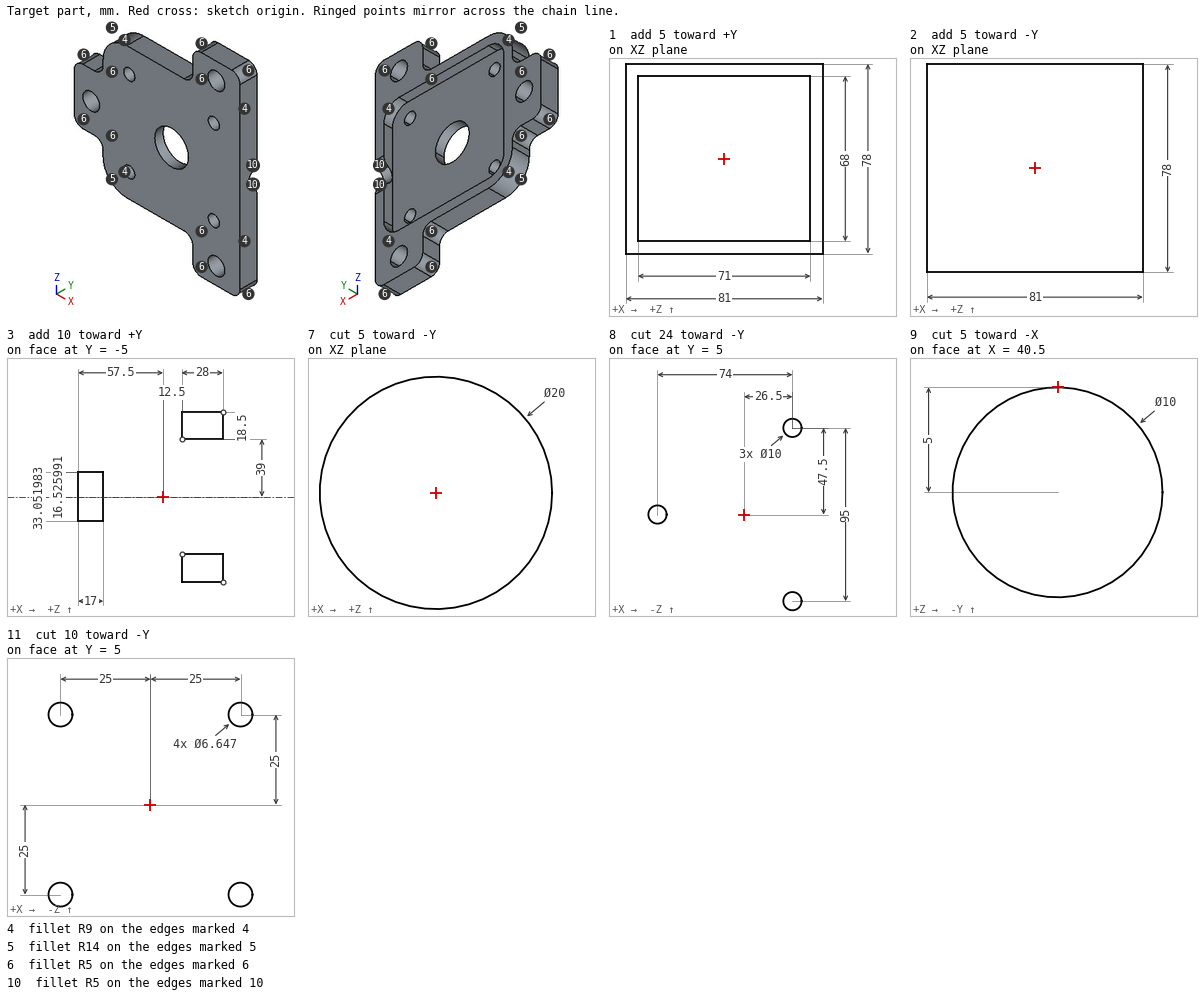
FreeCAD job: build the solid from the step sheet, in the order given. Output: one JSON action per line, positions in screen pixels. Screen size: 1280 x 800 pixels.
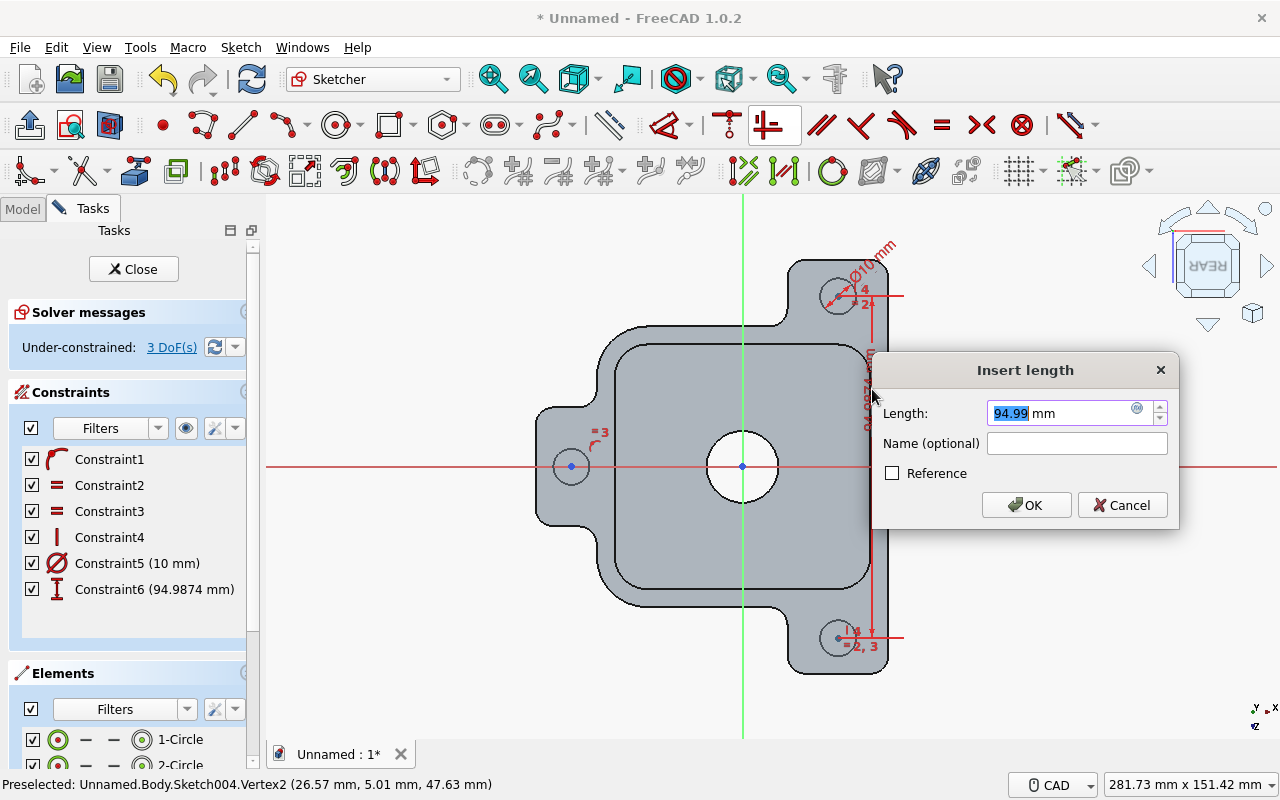
{"action": "type", "text": "95"}
{"action": "key", "text": "Return"}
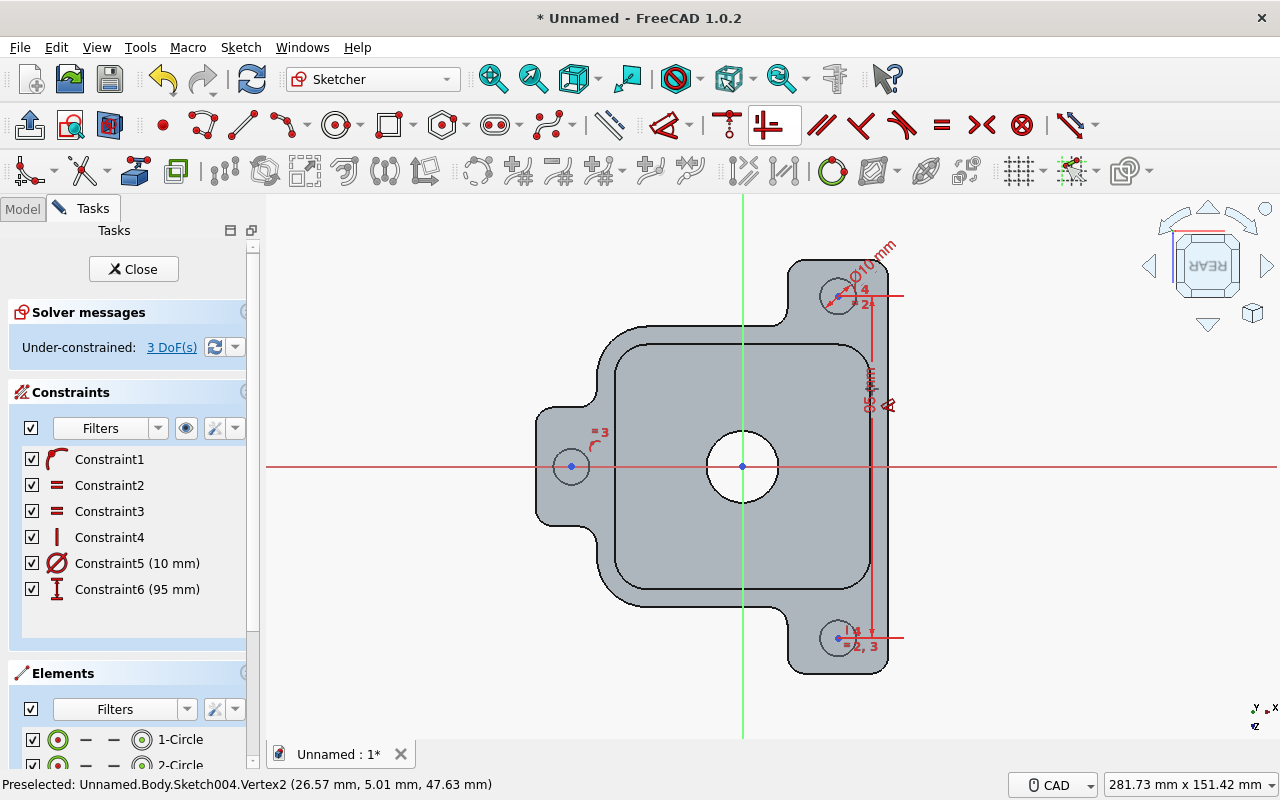
{"action": "left_click", "coordinate": [838, 296]}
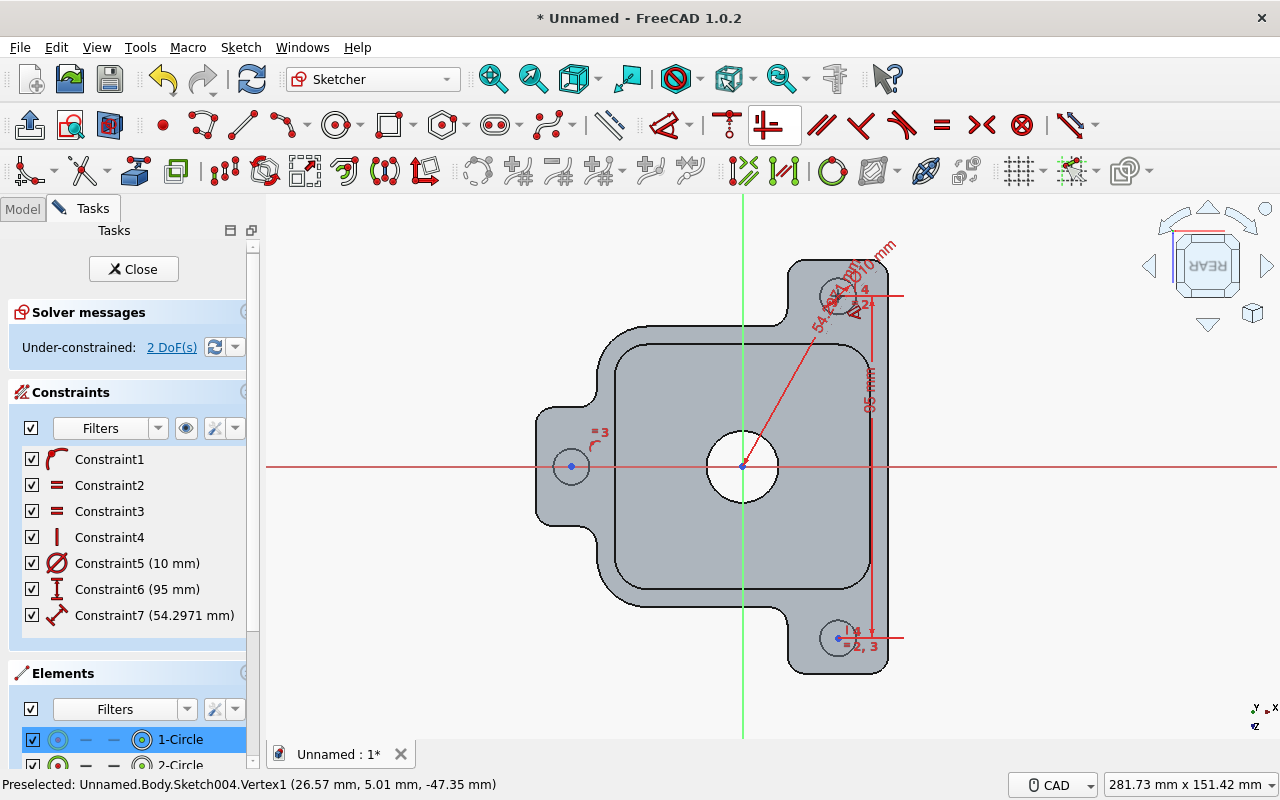
{"action": "left_click", "coordinate": [571, 467]}
{"action": "left_click", "coordinate": [705, 262]}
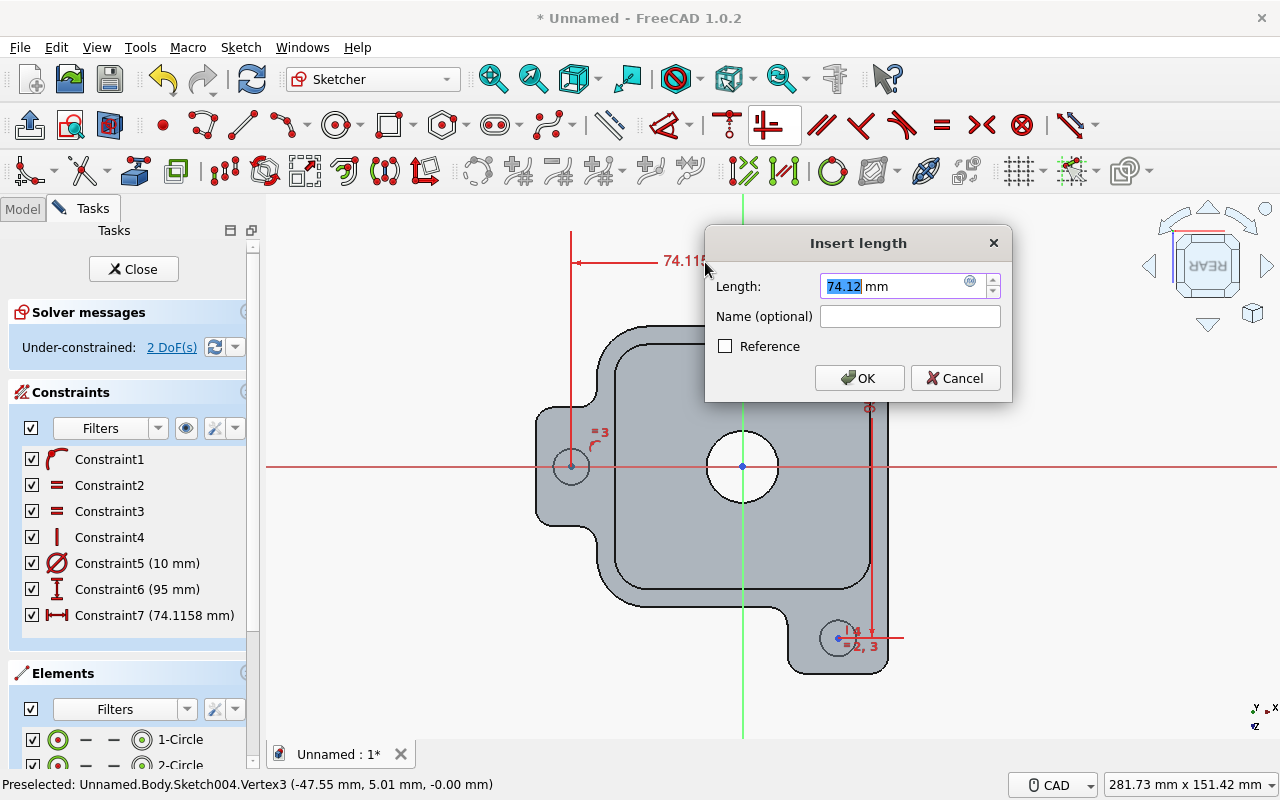
{"action": "type", "text": "74"}
{"action": "key", "text": "Return"}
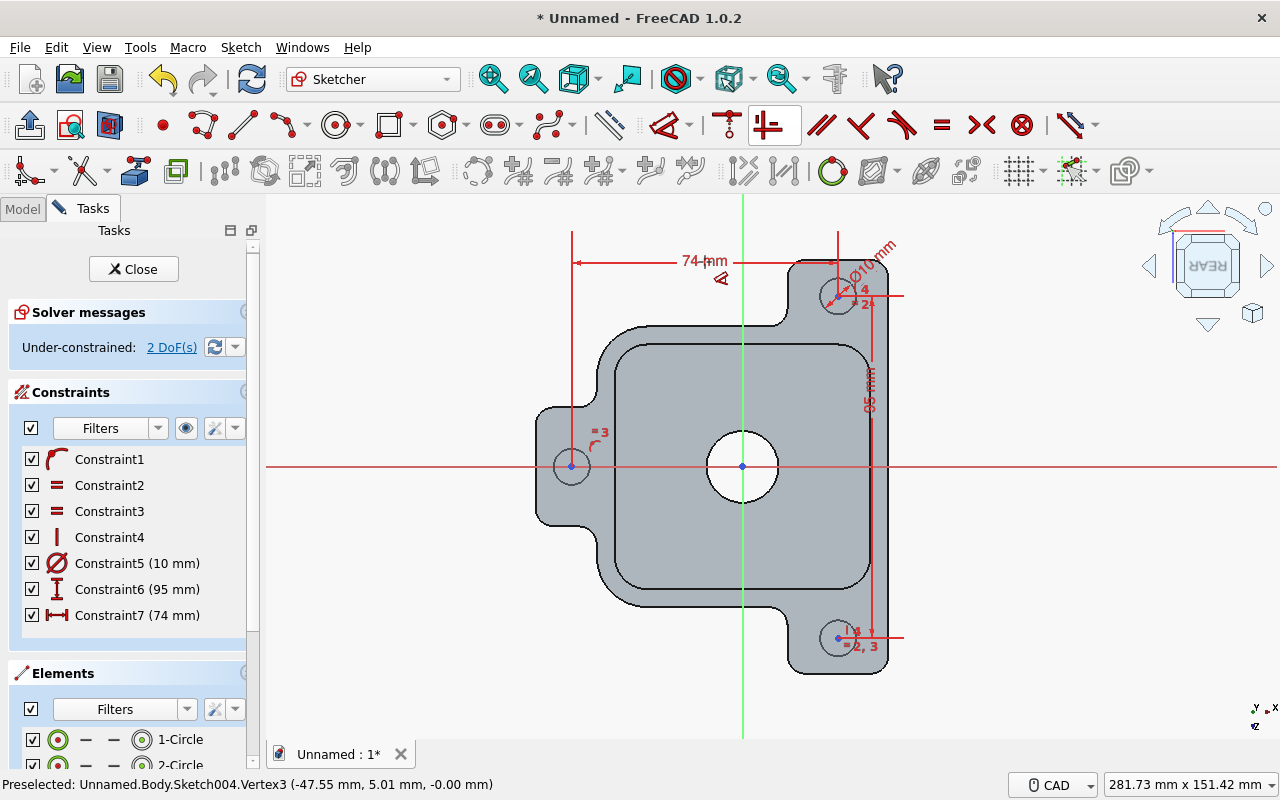
{"action": "left_click", "coordinate": [838, 296]}
{"action": "left_click", "coordinate": [790, 262]}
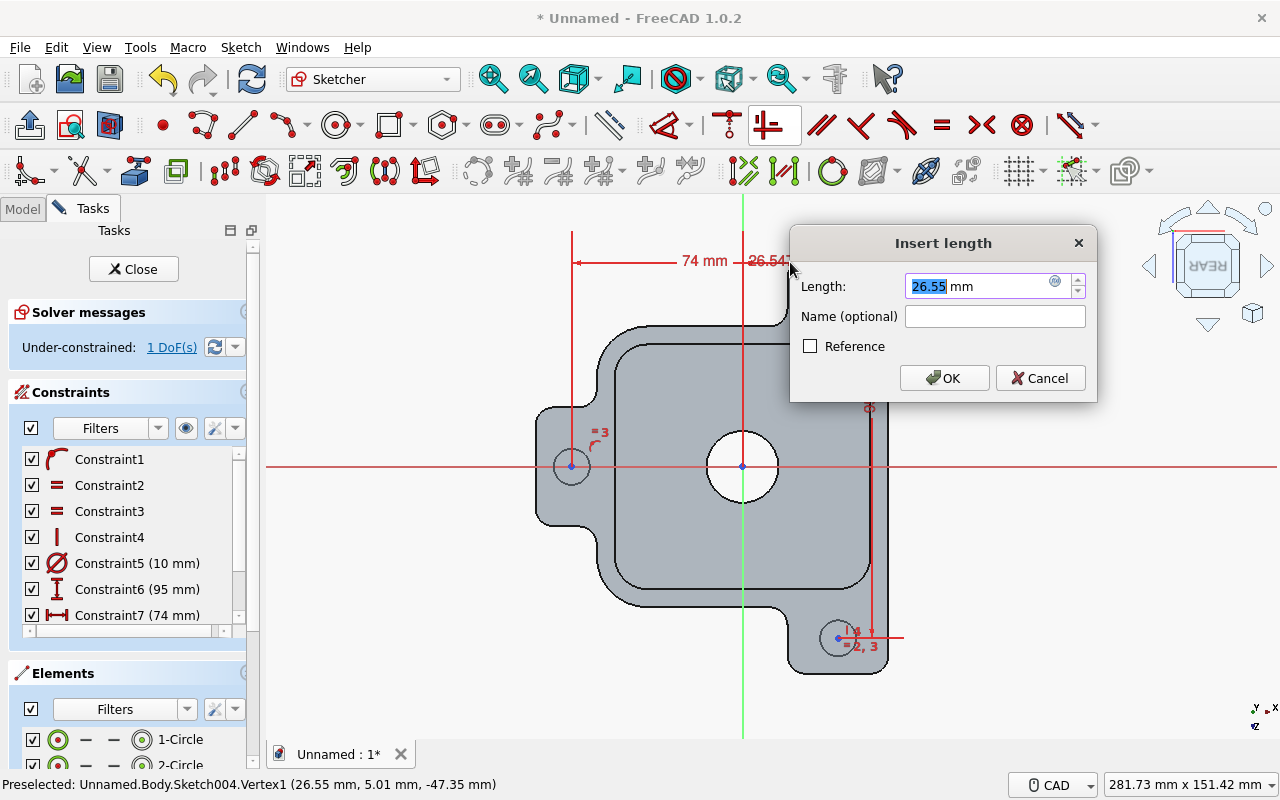
{"action": "type", "text": "26.5"}
{"action": "key", "text": "Return"}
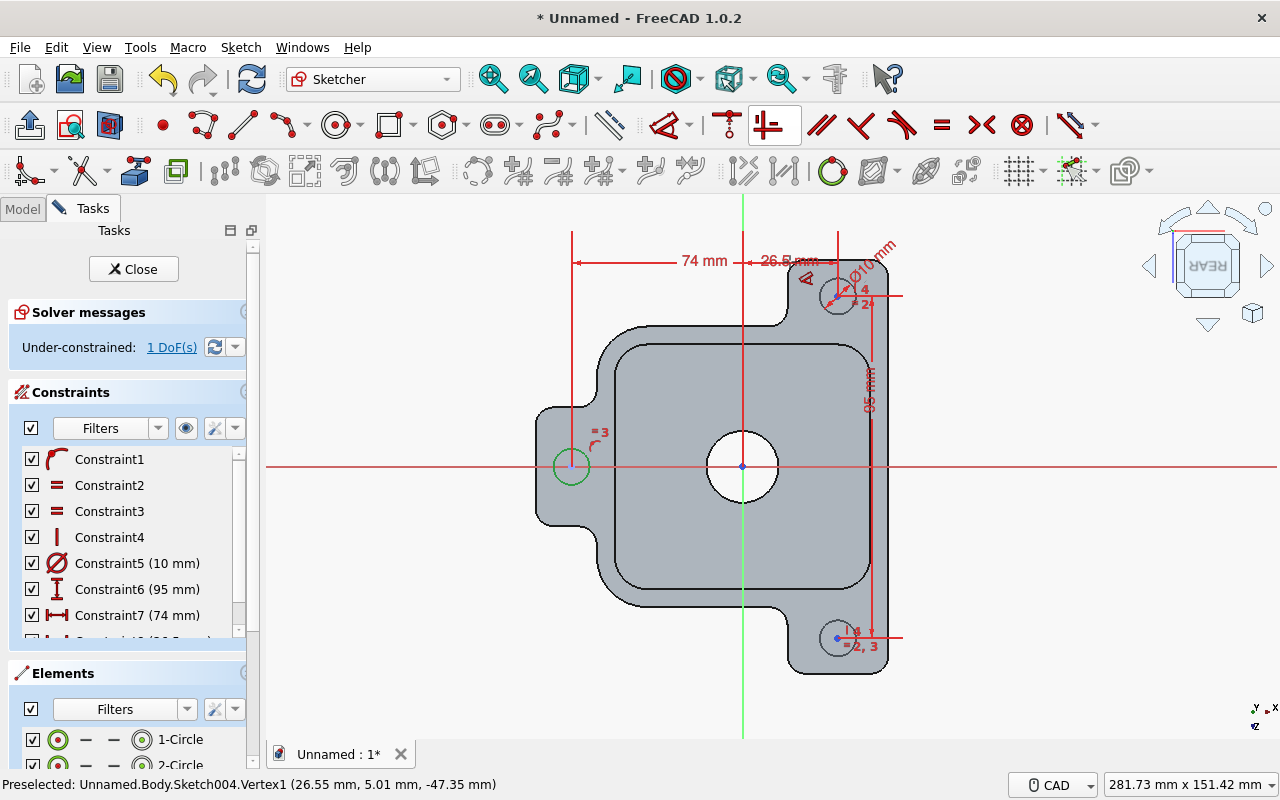
{"action": "left_click", "coordinate": [838, 296]}
{"action": "left_click", "coordinate": [872, 342]}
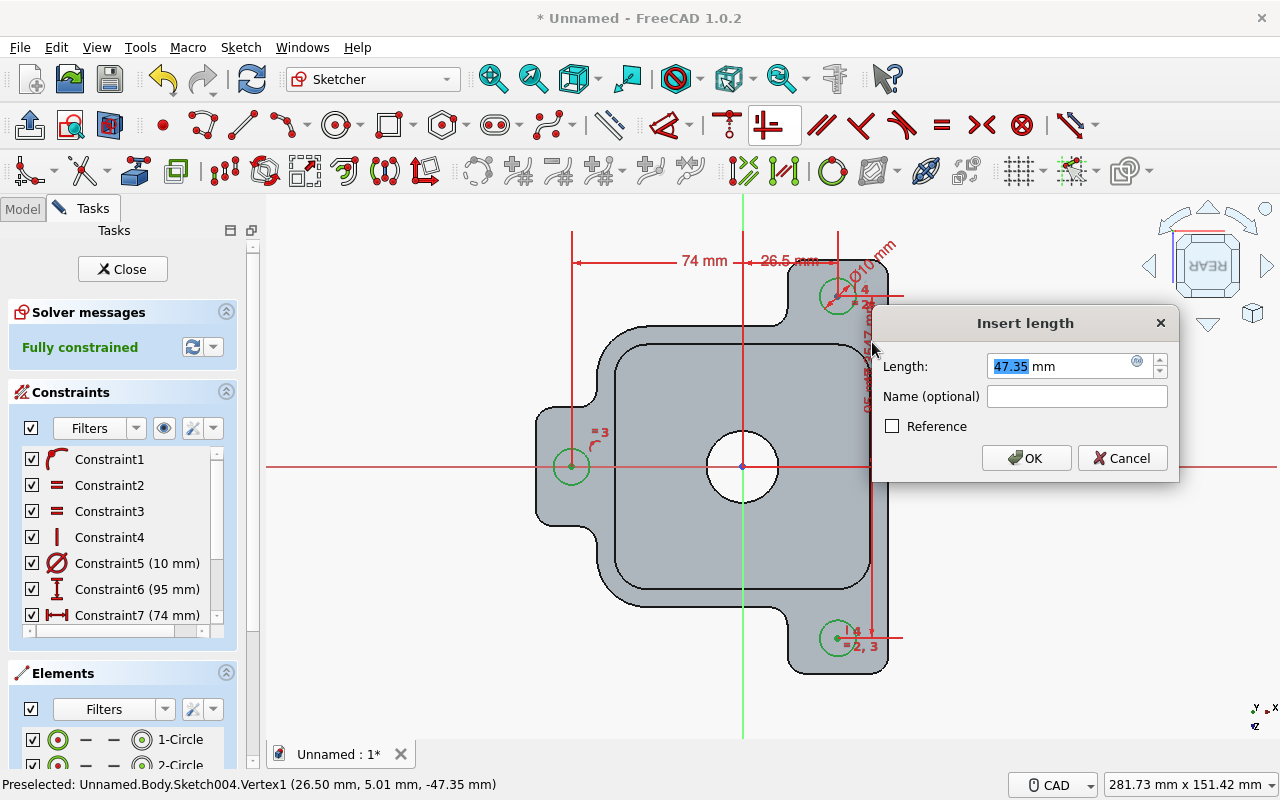
{"action": "type", "text": "47.5"}
{"action": "key", "text": "Return"}
{"action": "key", "text": "Escape"}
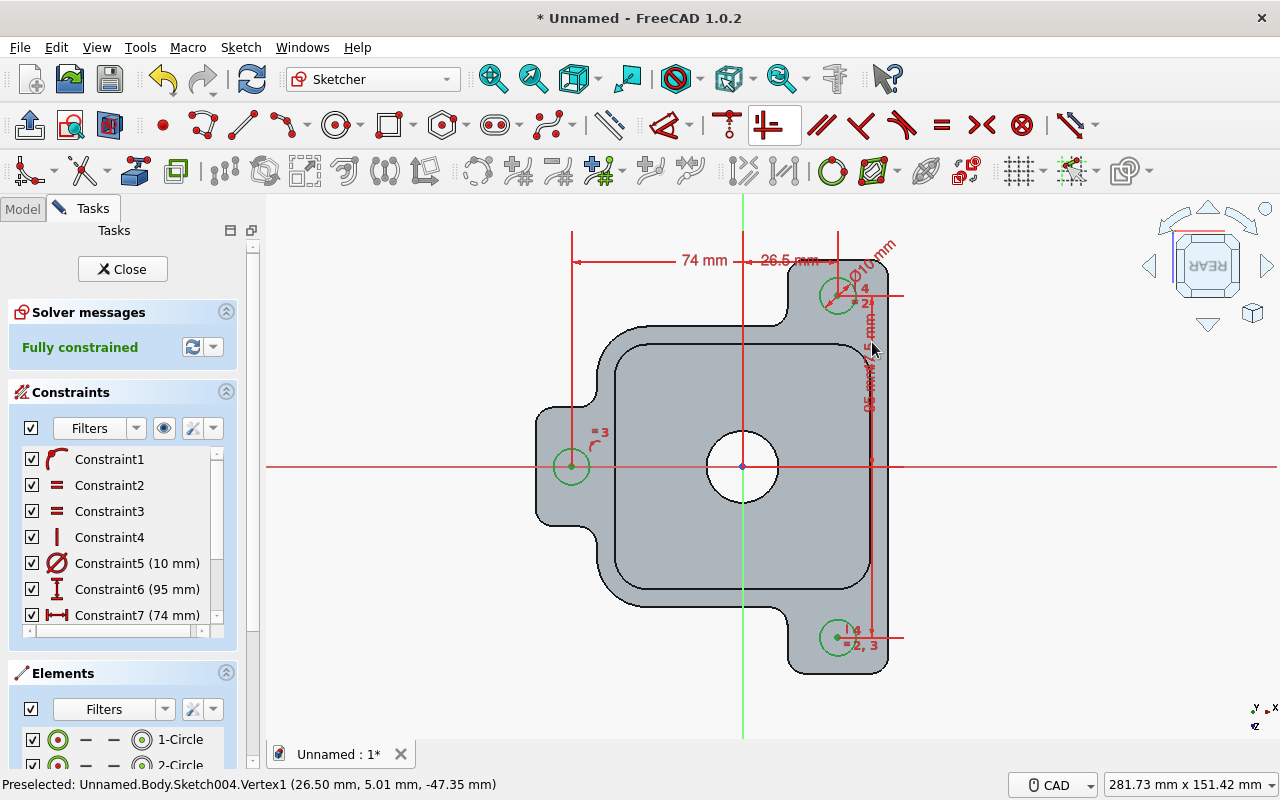
{"action": "left_click", "coordinate": [123, 269]}